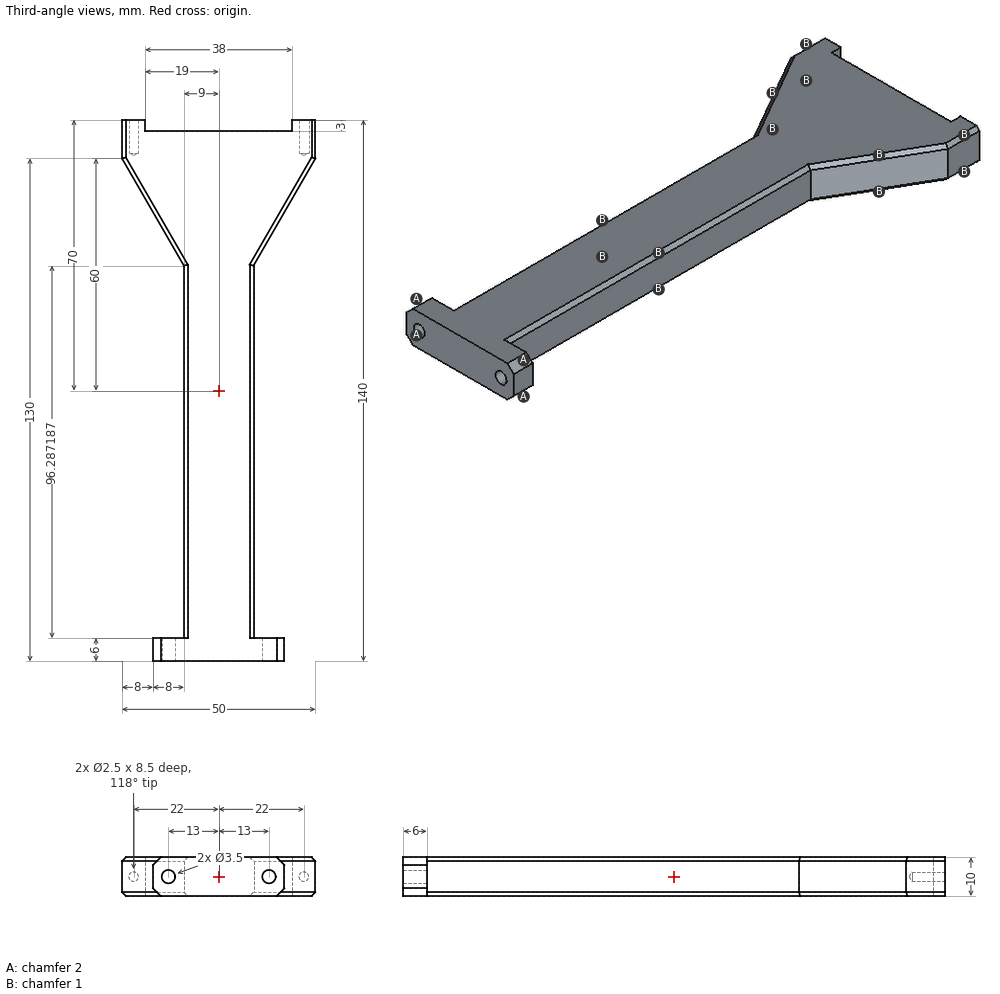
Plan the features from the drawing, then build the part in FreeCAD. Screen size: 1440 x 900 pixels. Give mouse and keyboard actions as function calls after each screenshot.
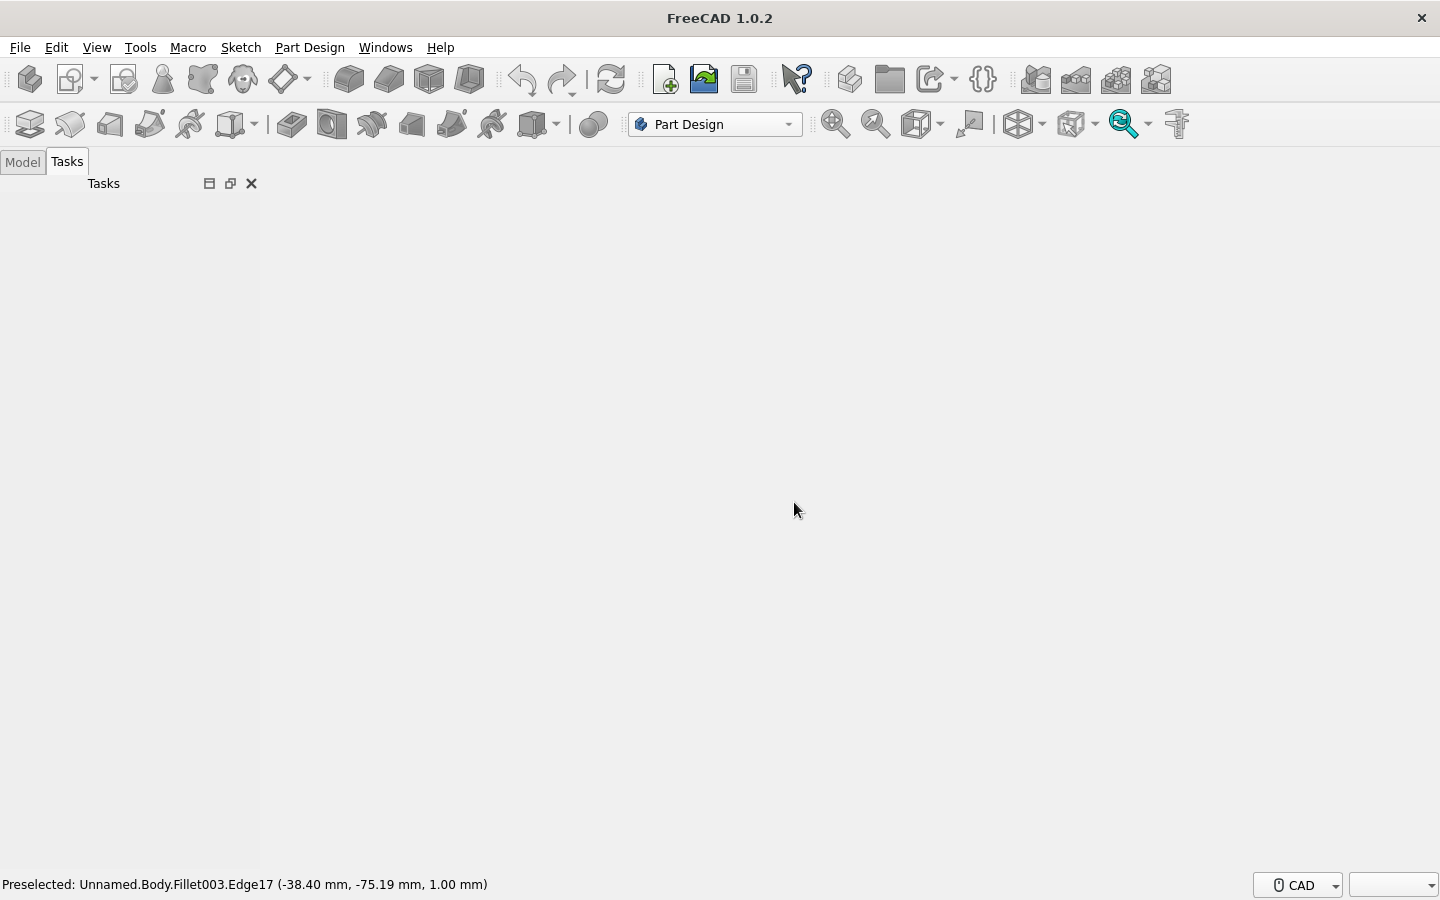
click(664, 80)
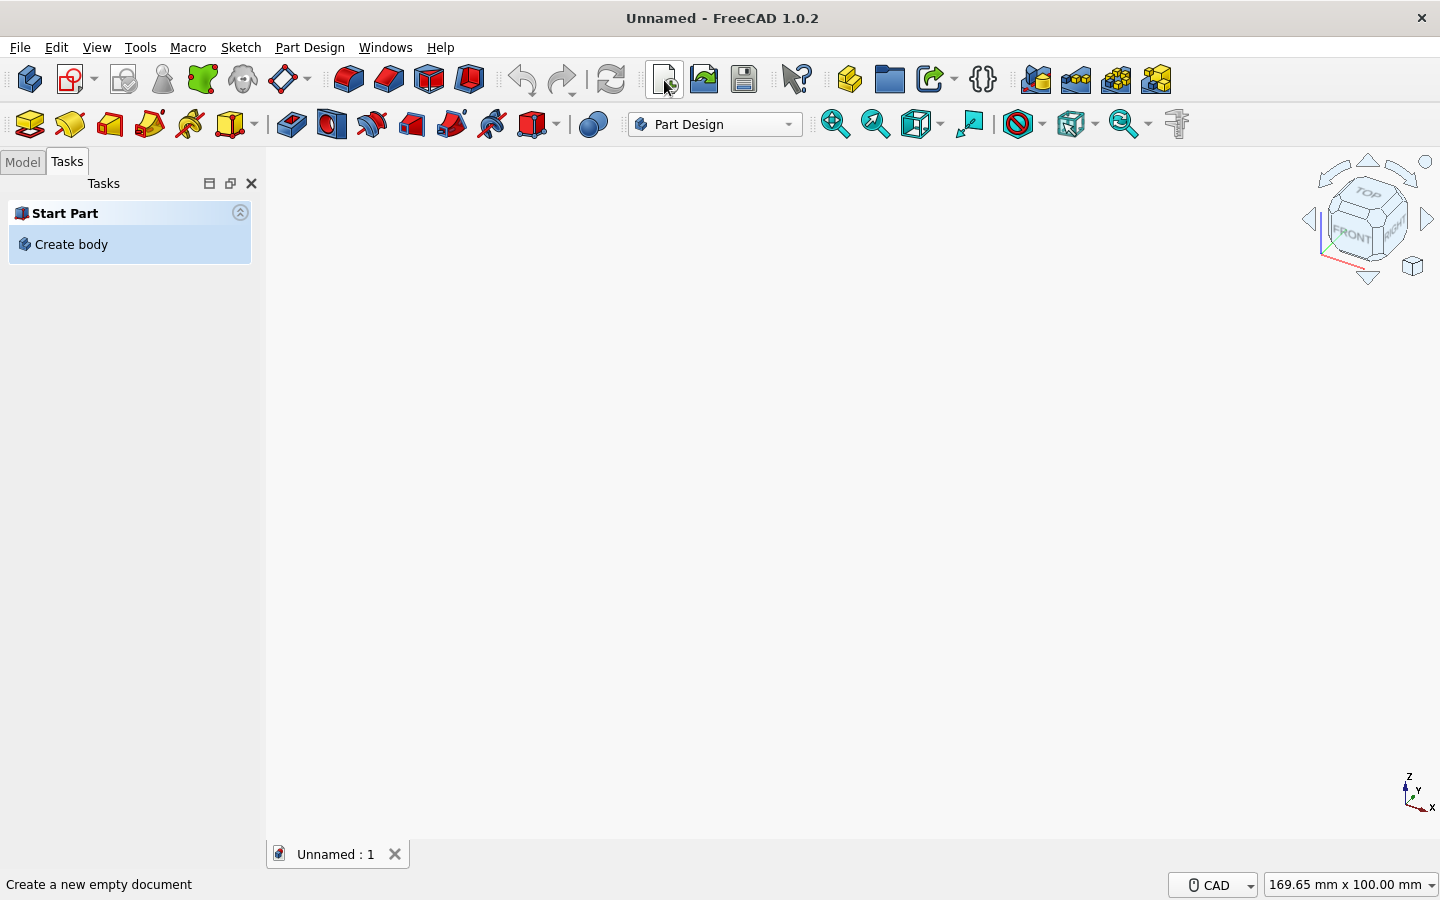
click(70, 80)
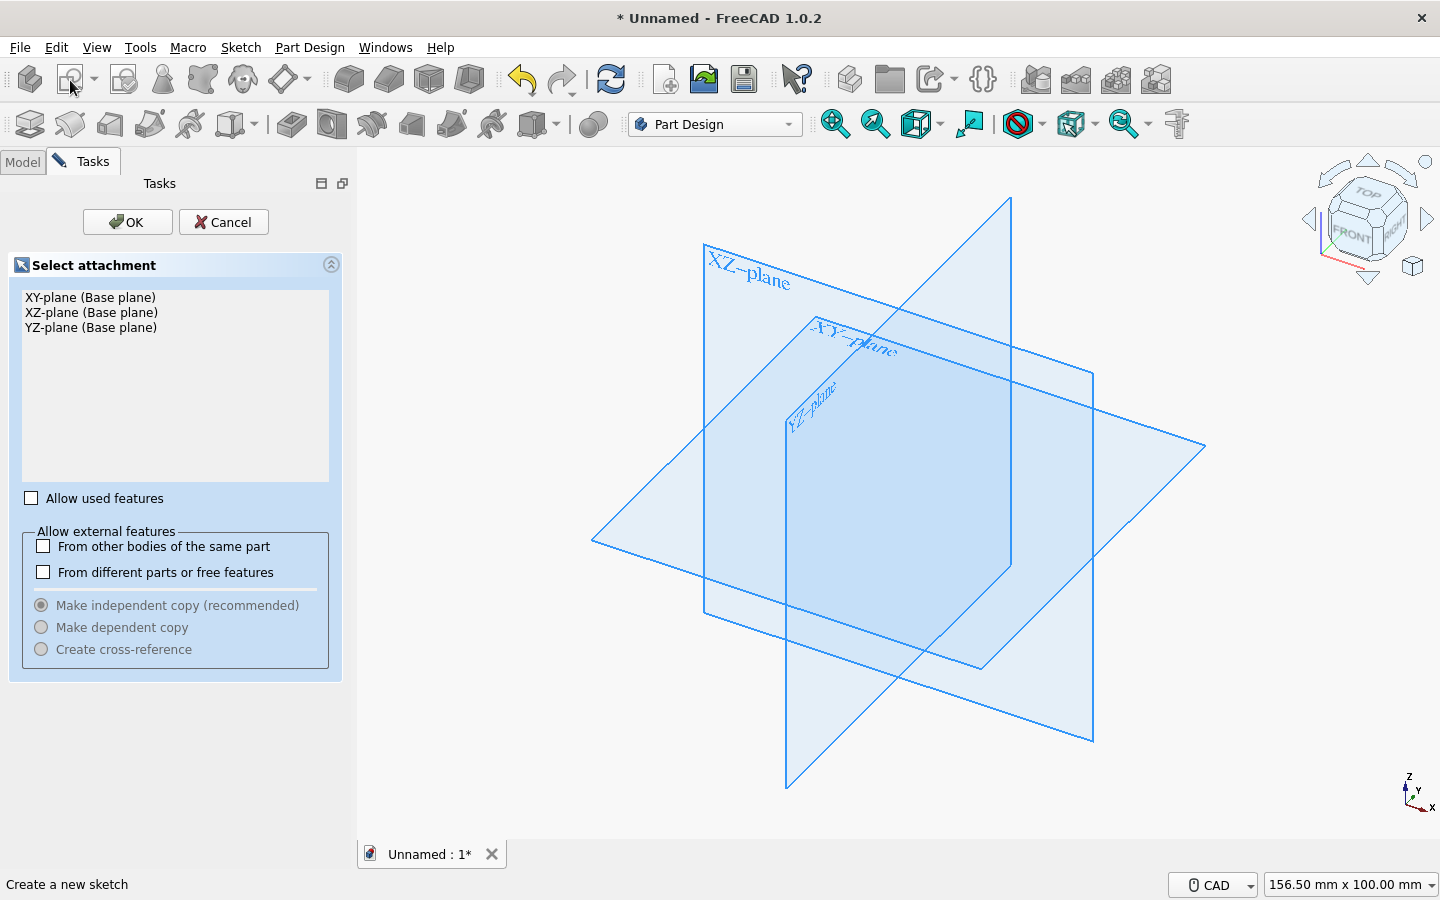
click(82, 298)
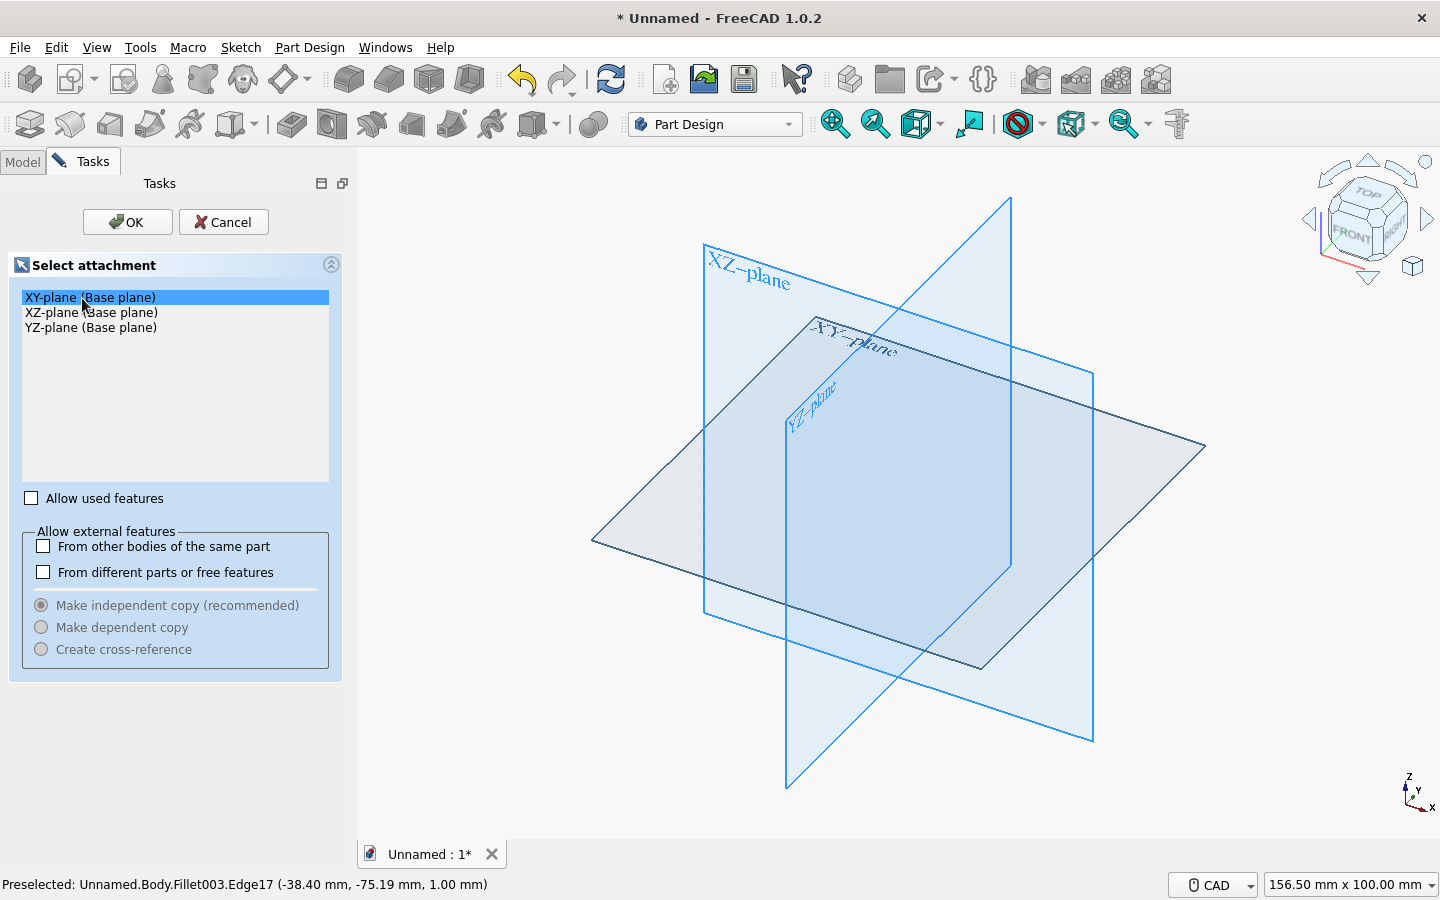
click(128, 222)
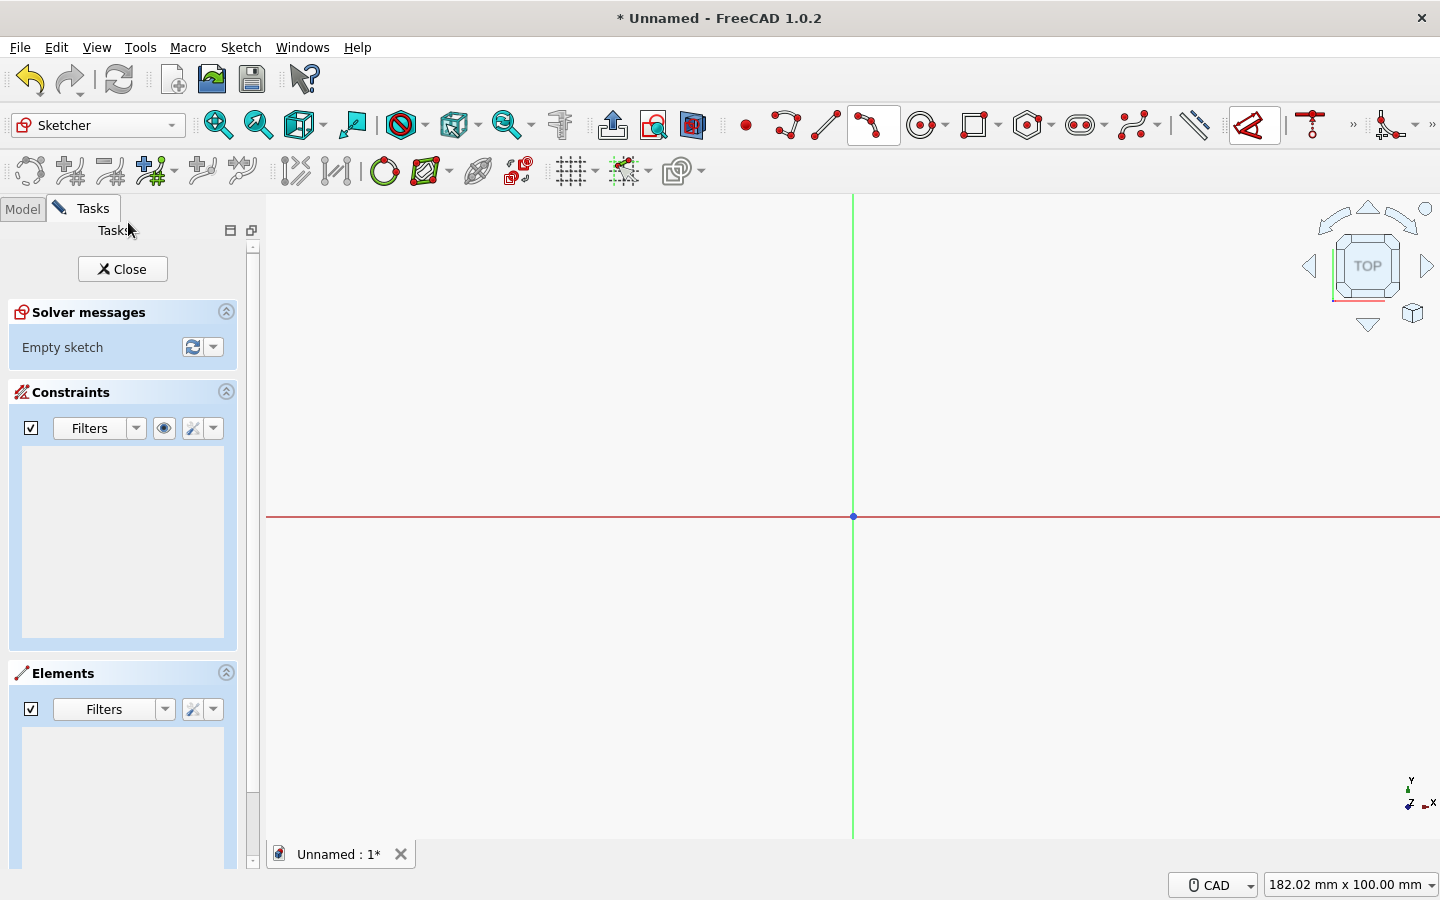
scroll(729, 516, down, 4)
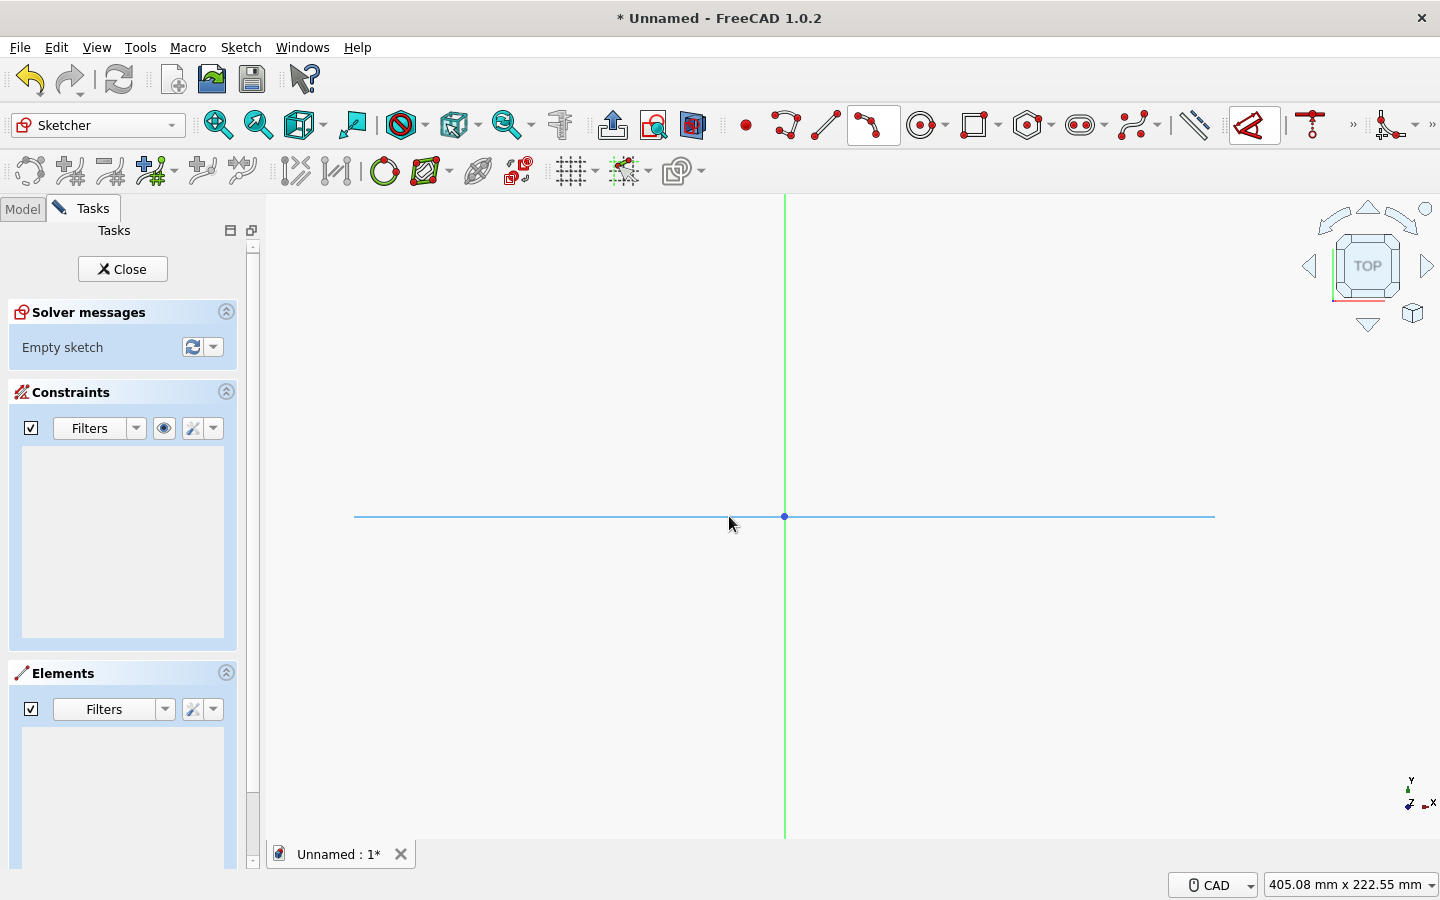
click(1000, 126)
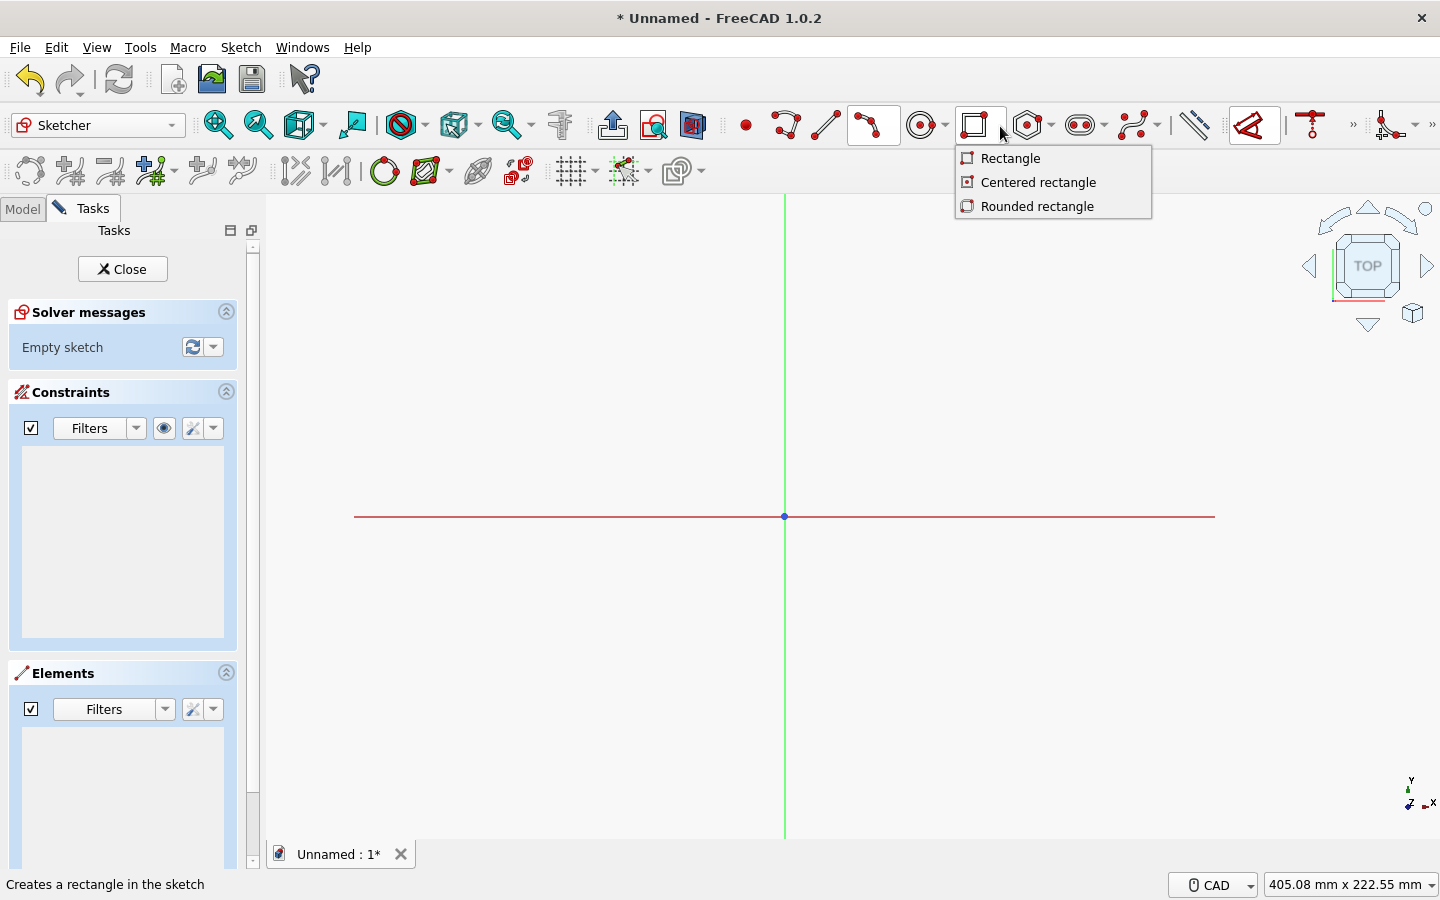
click(1054, 182)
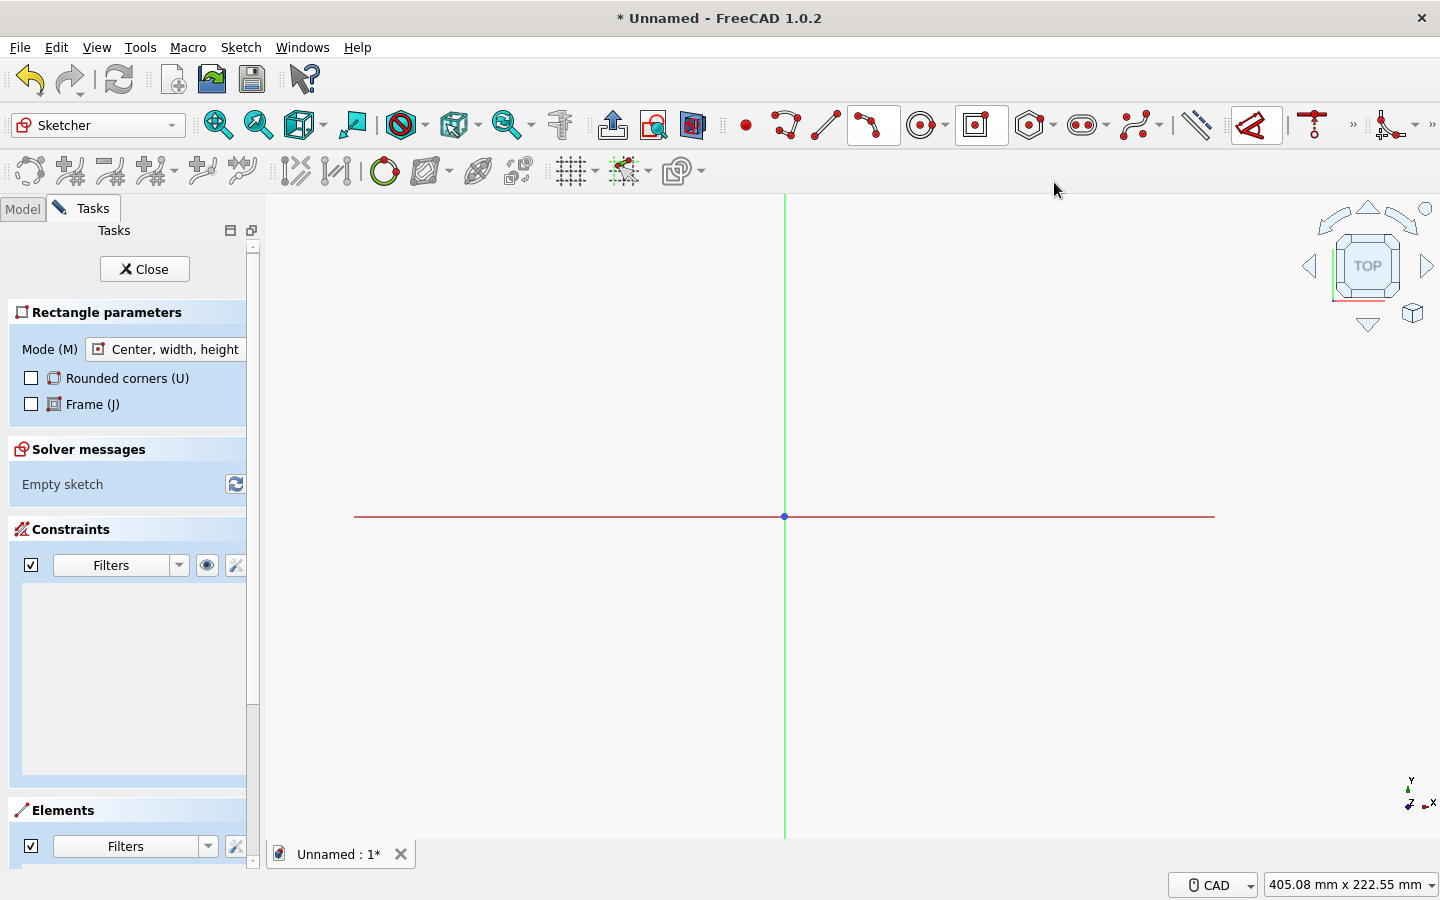
click(785, 516)
move(857, 314)